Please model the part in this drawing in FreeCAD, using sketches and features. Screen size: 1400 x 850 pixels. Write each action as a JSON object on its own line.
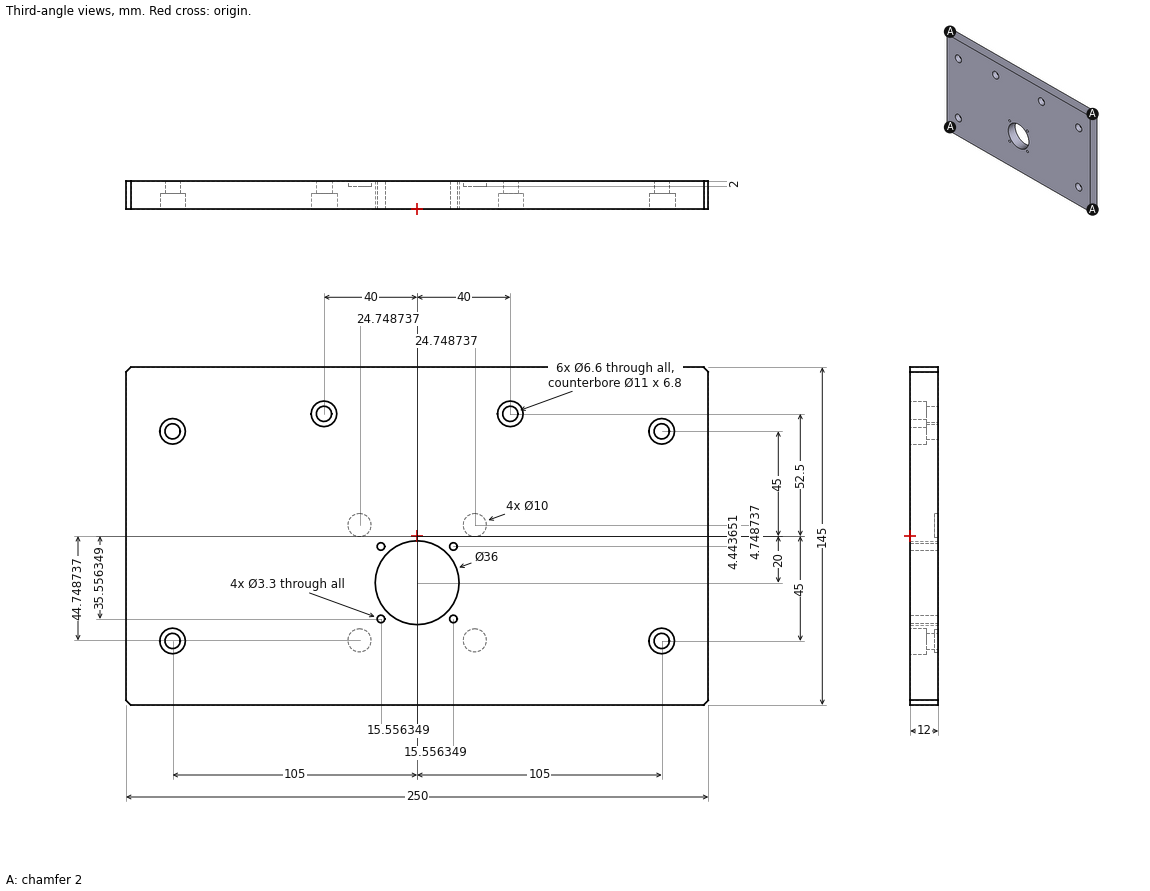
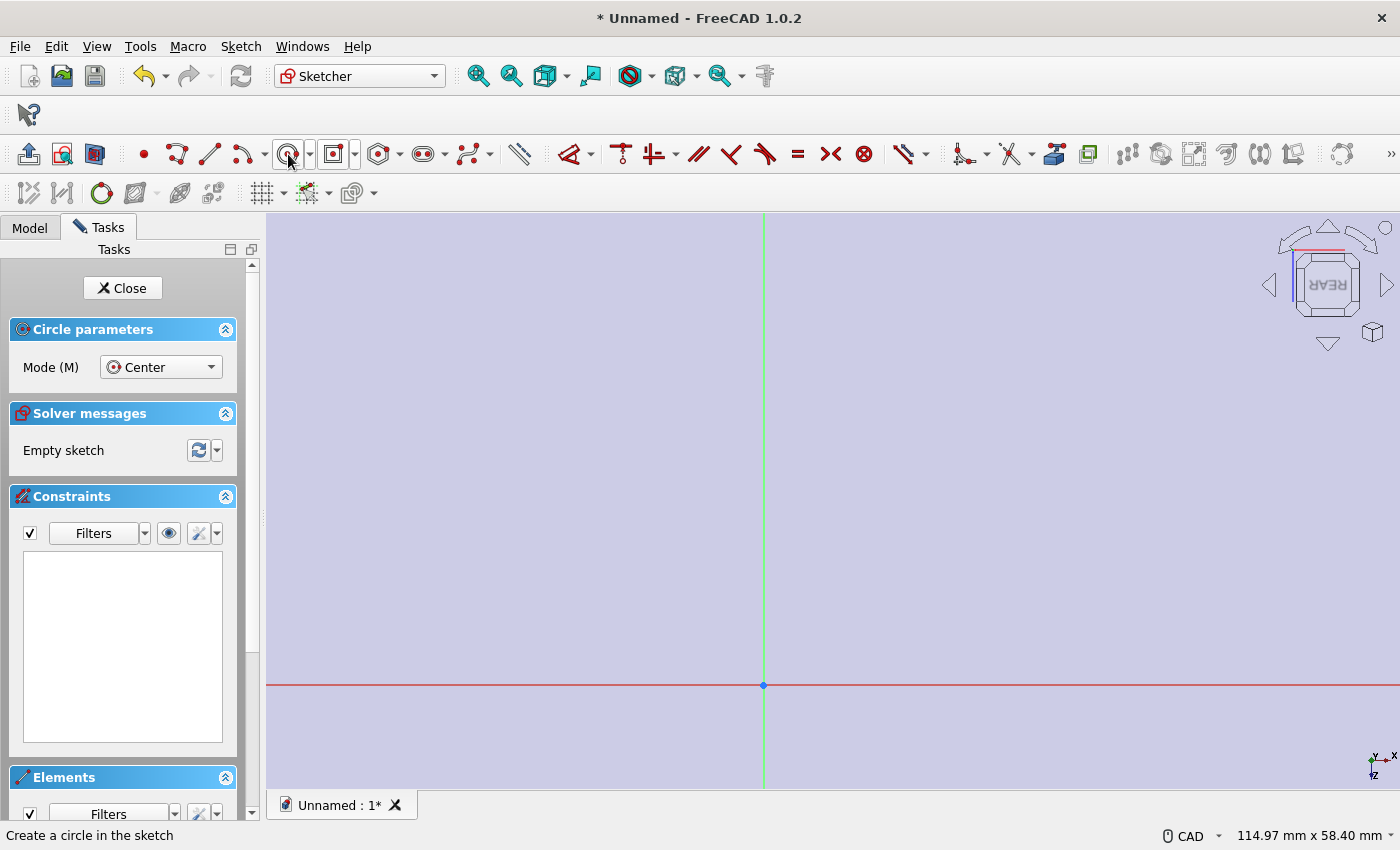
{"action": "left_click", "coordinate": [764, 488]}
{"action": "mouse_move", "coordinate": [889, 362]}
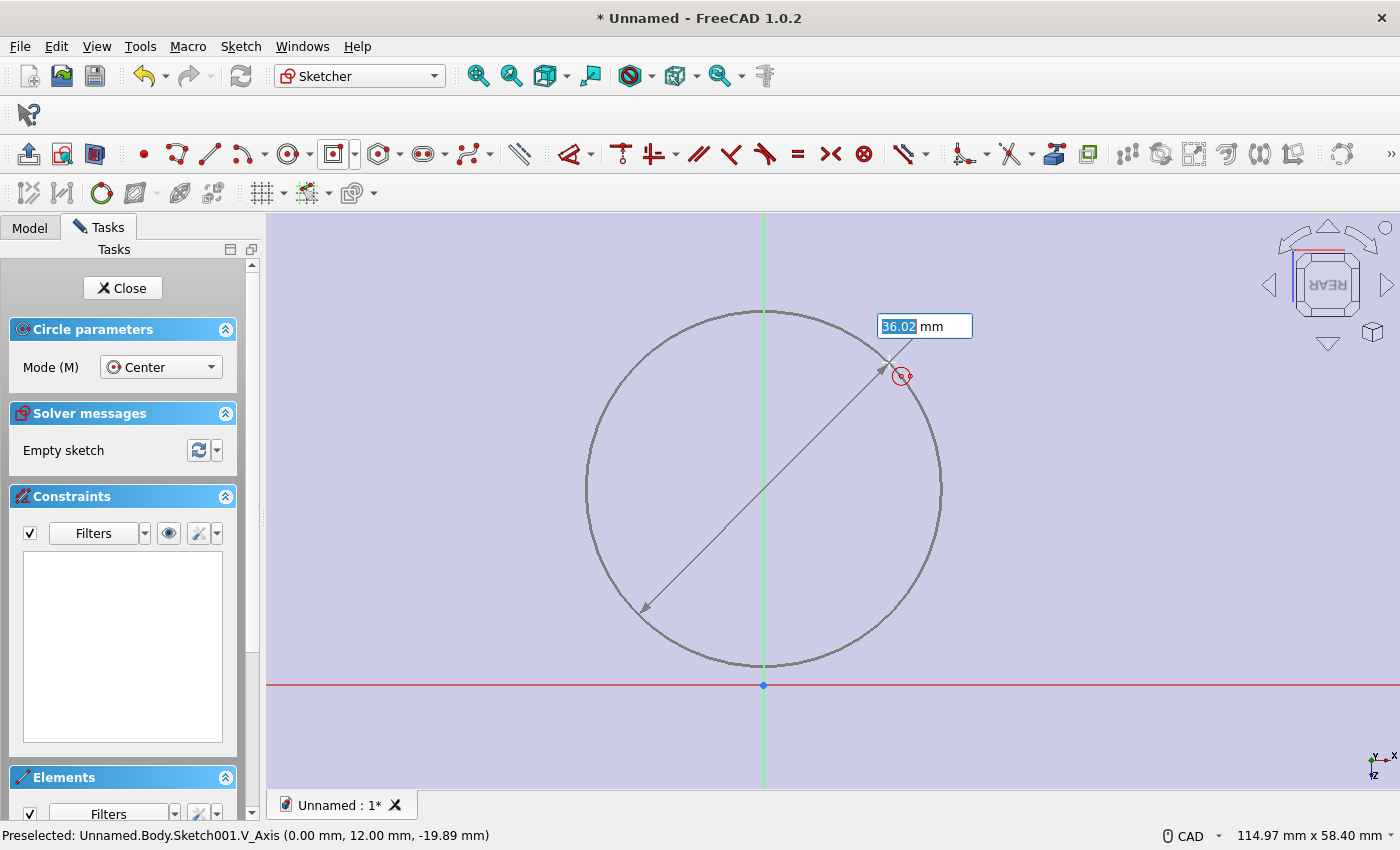
{"action": "type", "text": "36"}
{"action": "key", "text": "Return"}
{"action": "key", "text": "Escape"}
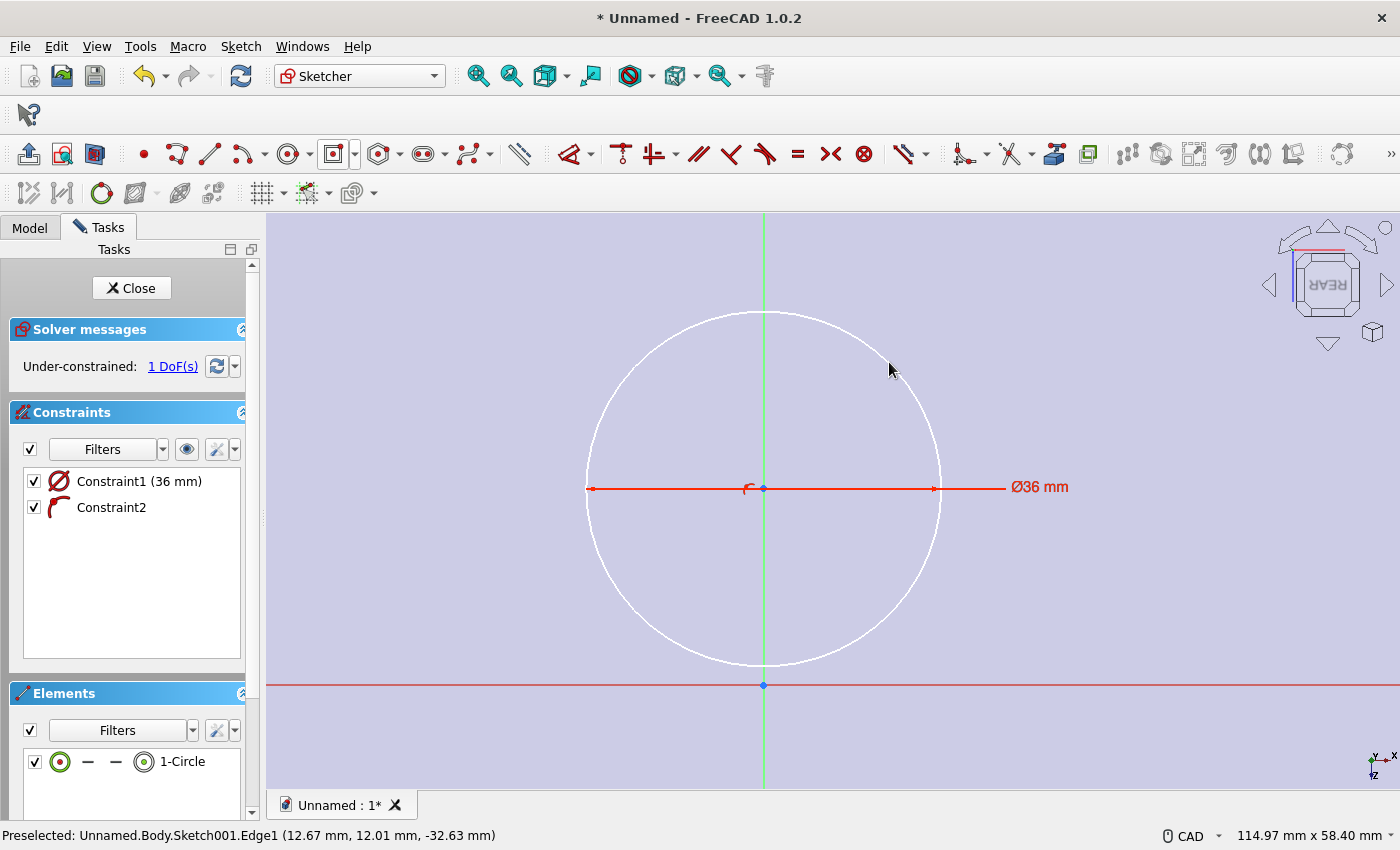
{"action": "left_click", "coordinate": [568, 154]}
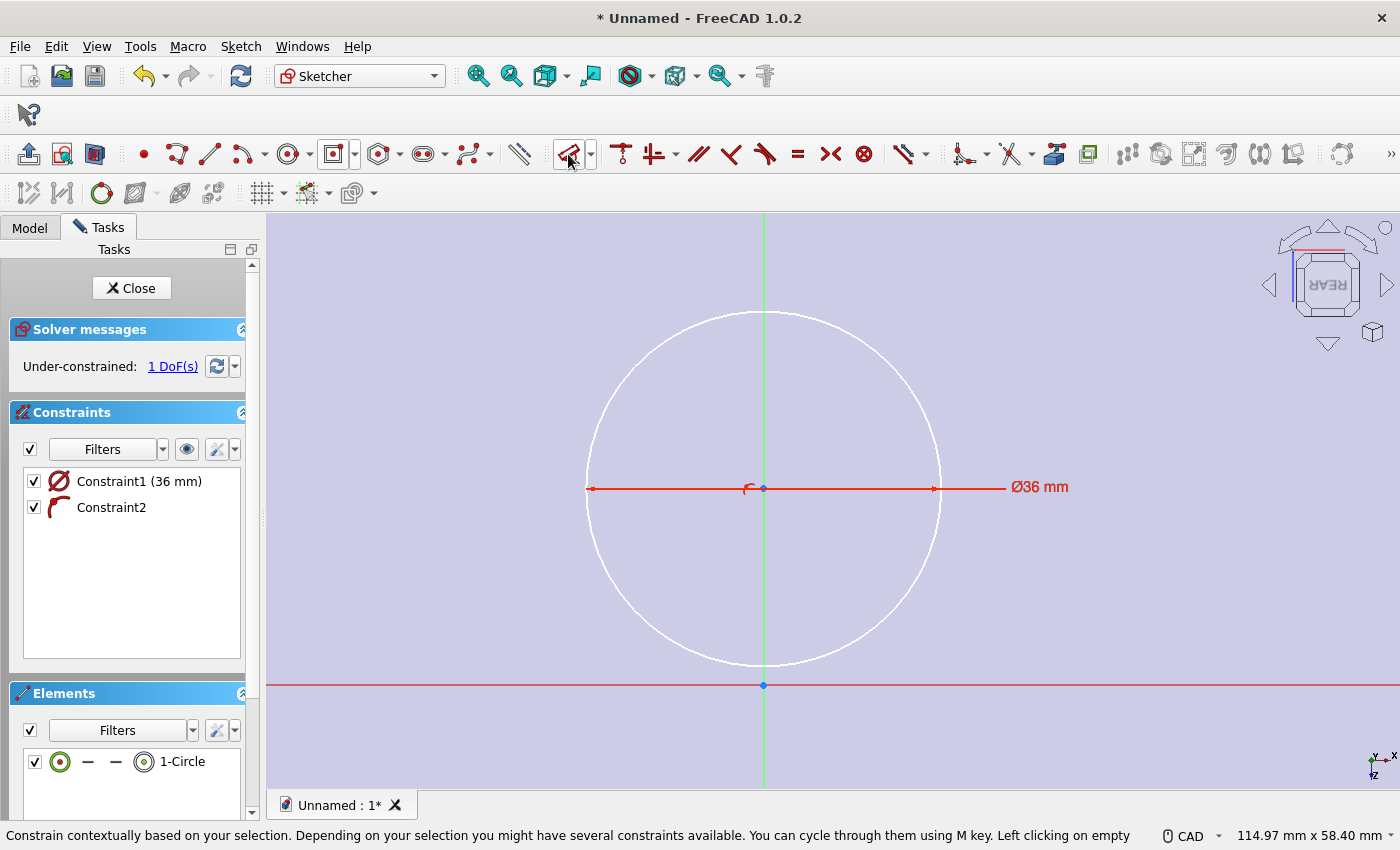
{"action": "left_click", "coordinate": [764, 489]}
{"action": "left_click", "coordinate": [798, 587]}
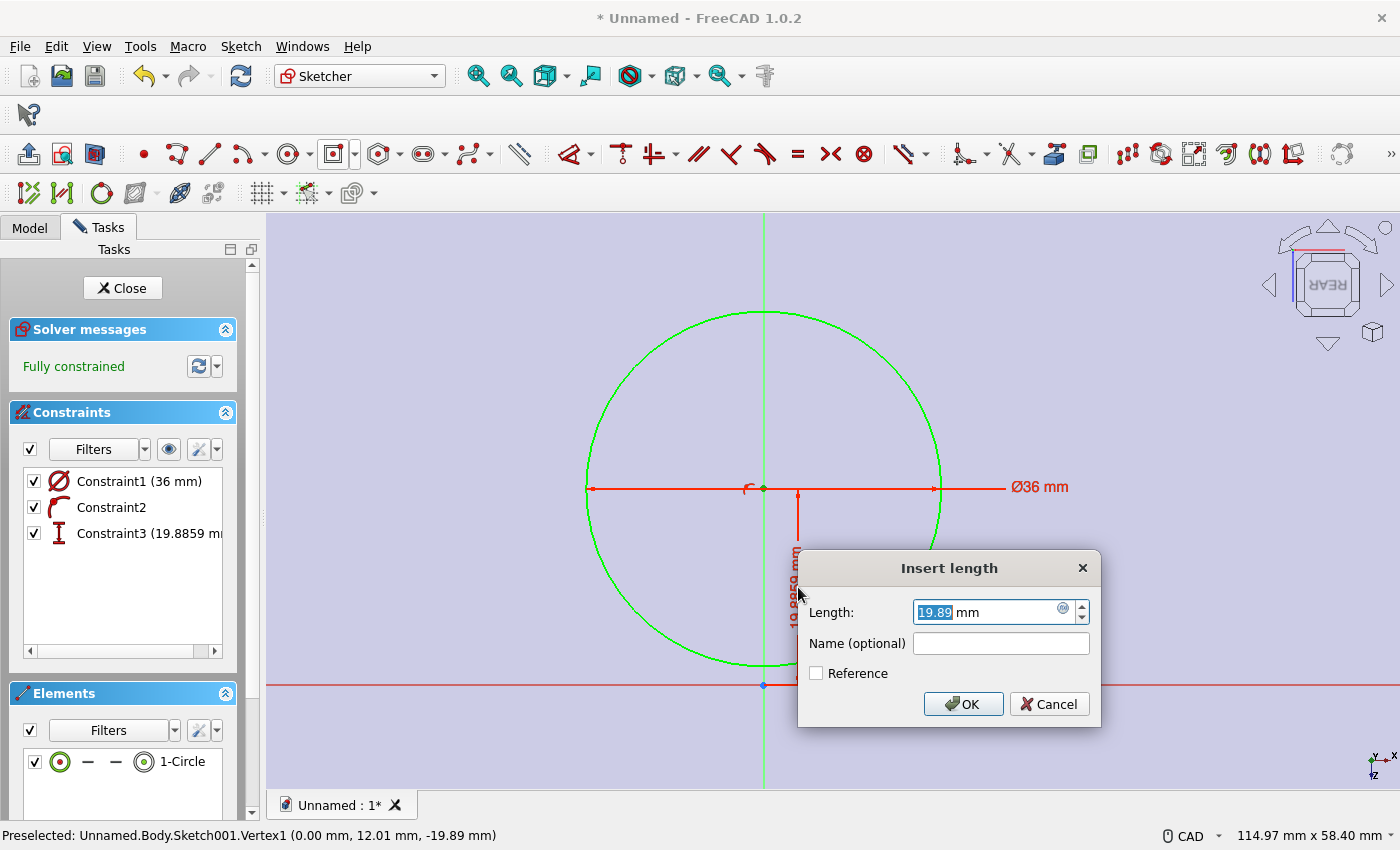
{"action": "type", "text": "20"}
{"action": "key", "text": "Return"}
{"action": "key", "text": "Escape"}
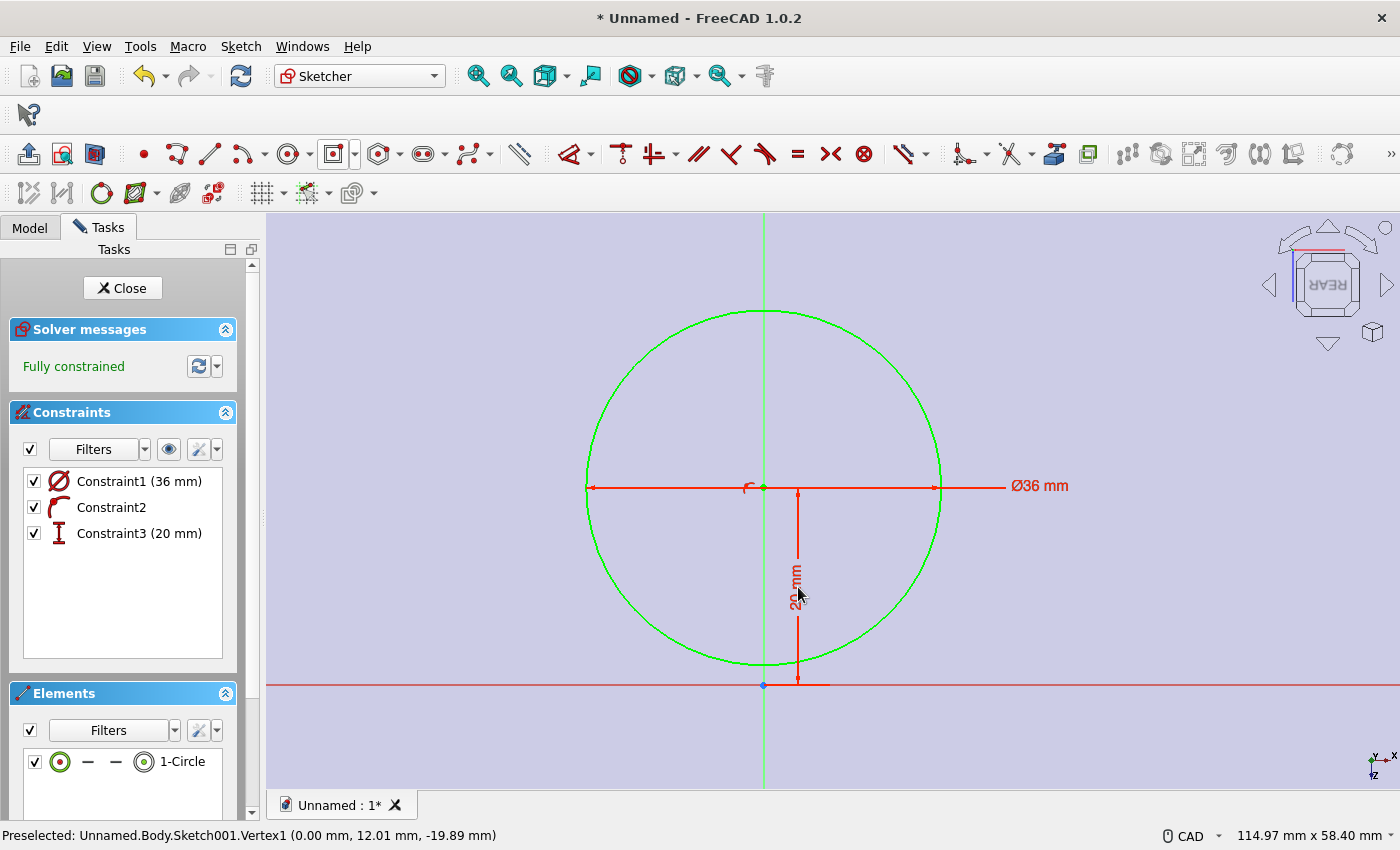
{"action": "left_click", "coordinate": [123, 288]}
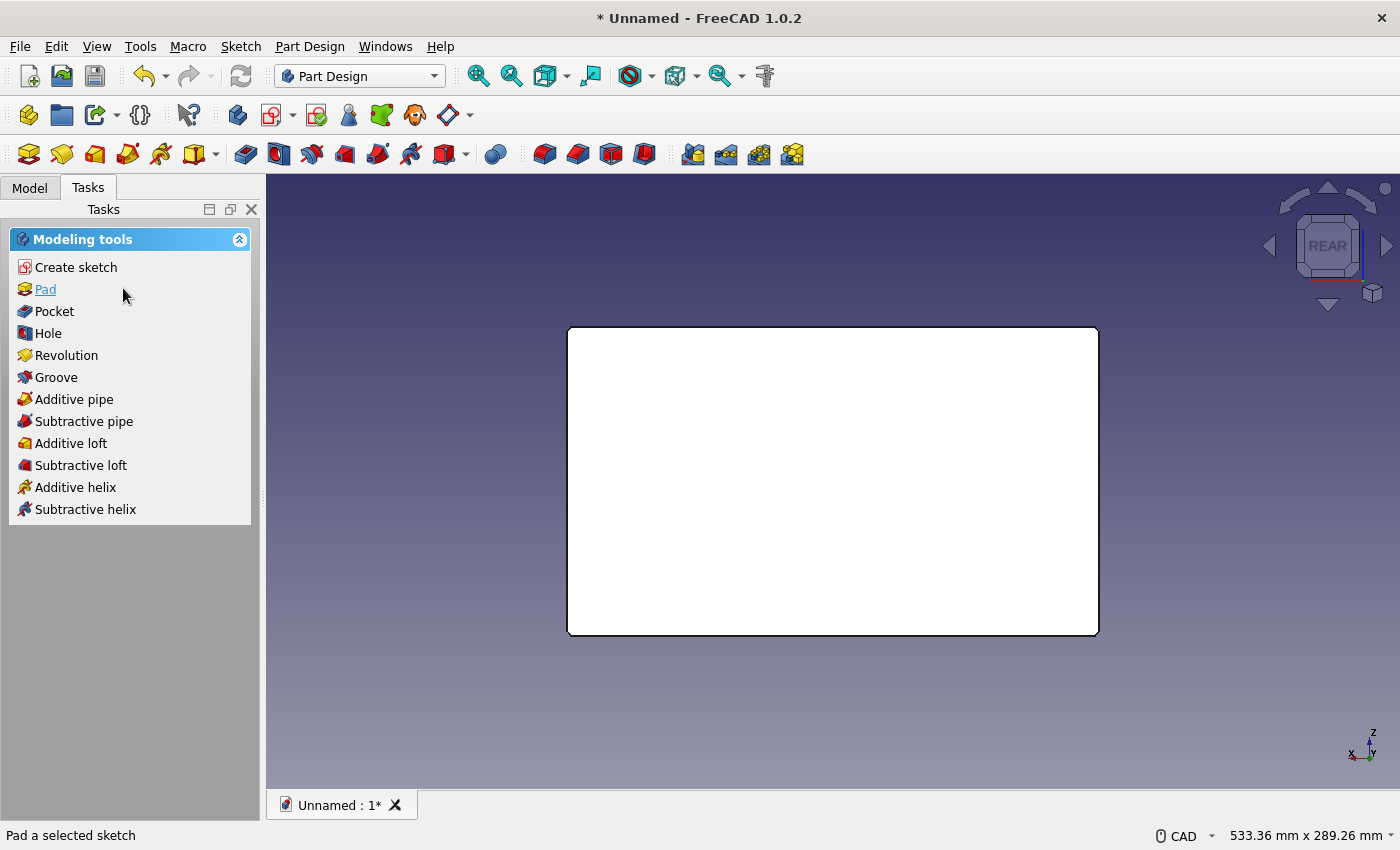
{"action": "left_click", "coordinate": [246, 154]}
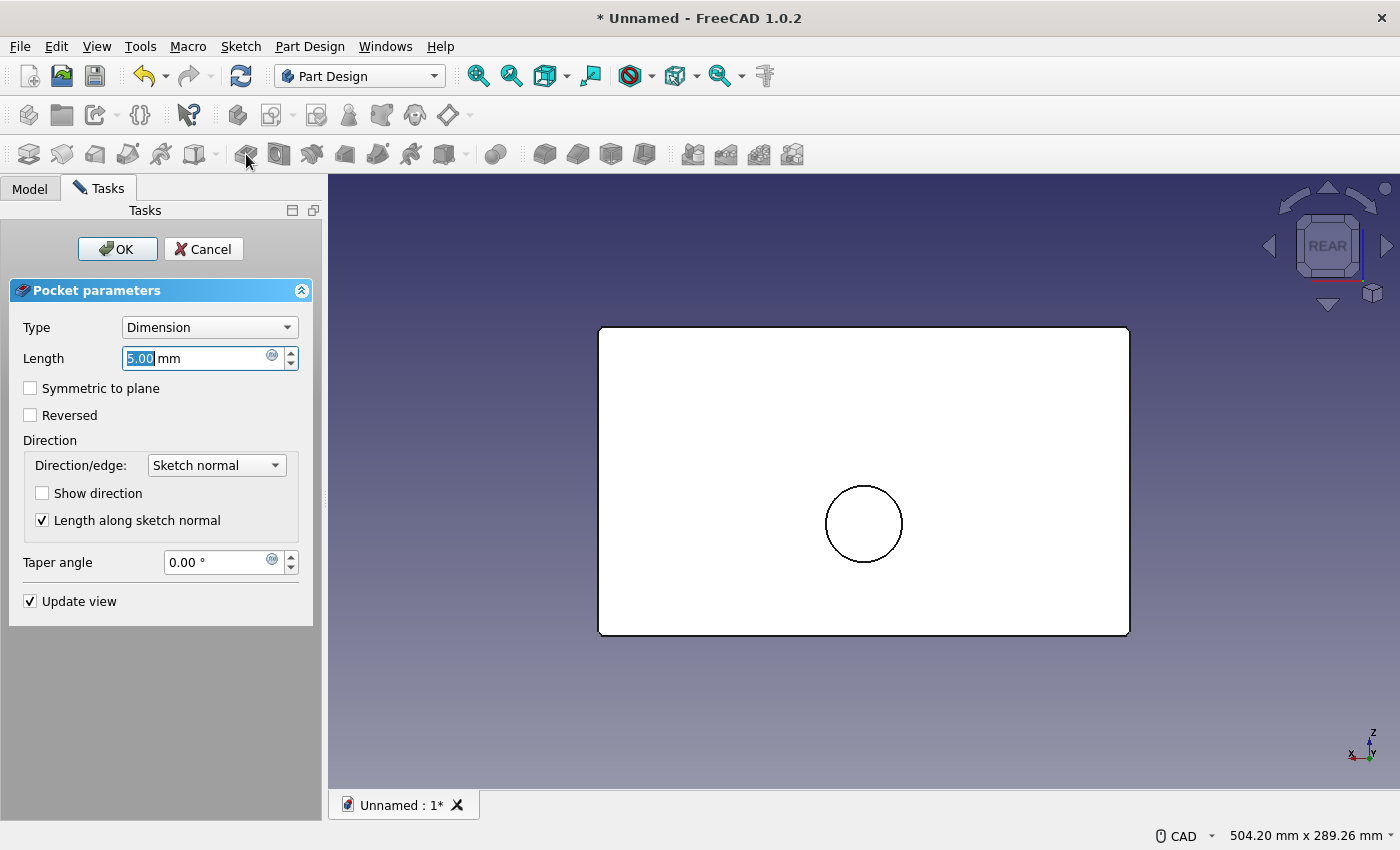
{"action": "left_click", "coordinate": [210, 328]}